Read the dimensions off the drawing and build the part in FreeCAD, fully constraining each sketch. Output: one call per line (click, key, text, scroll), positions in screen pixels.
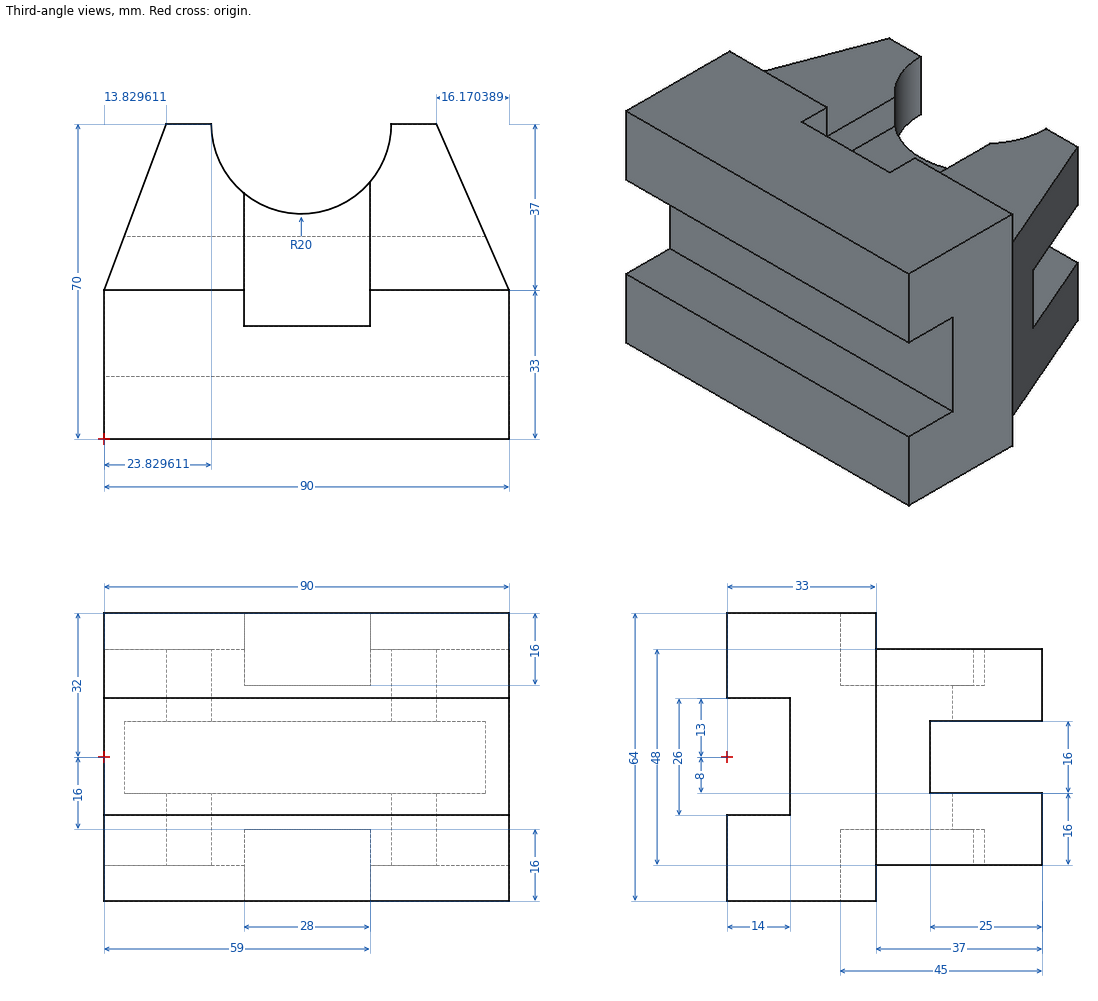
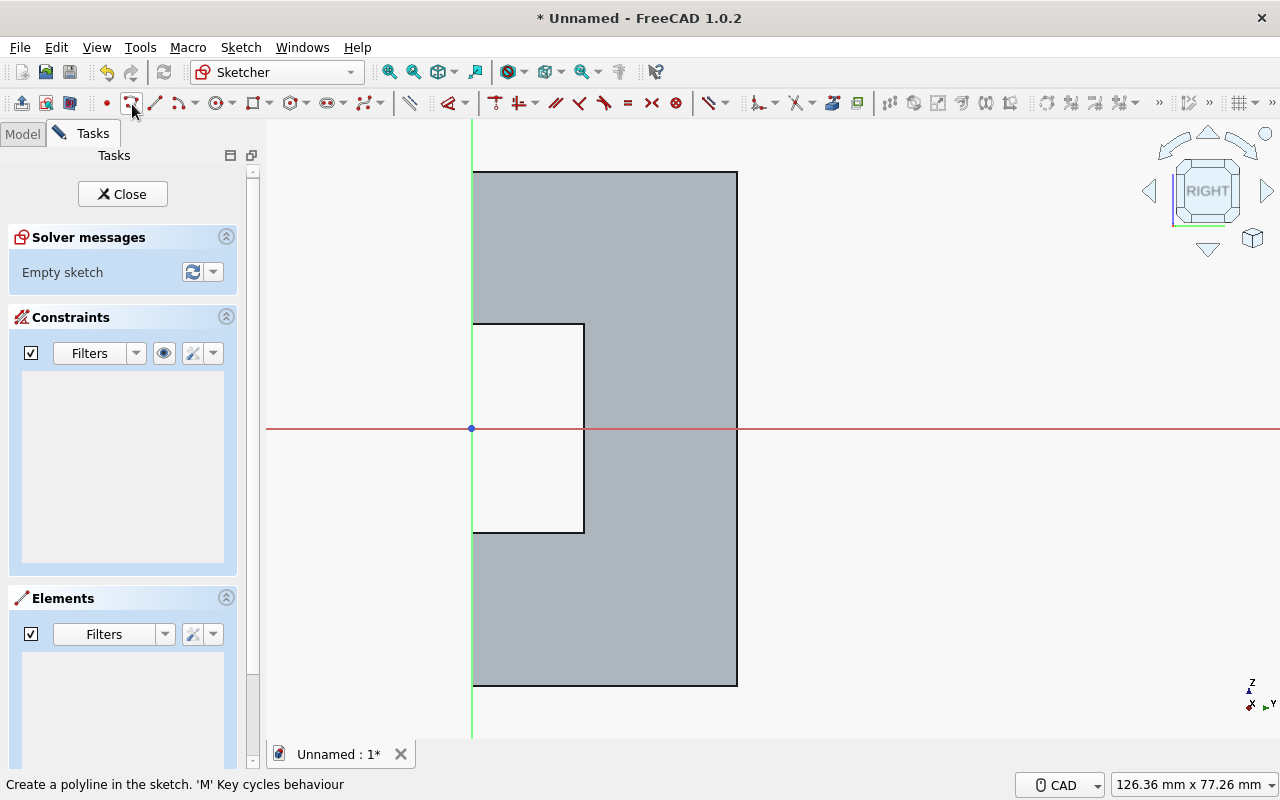
click(737, 236)
click(737, 621)
click(1034, 621)
click(1034, 493)
click(833, 493)
click(833, 365)
click(1034, 365)
click(1034, 236)
click(737, 237)
key(Escape)
key(Escape)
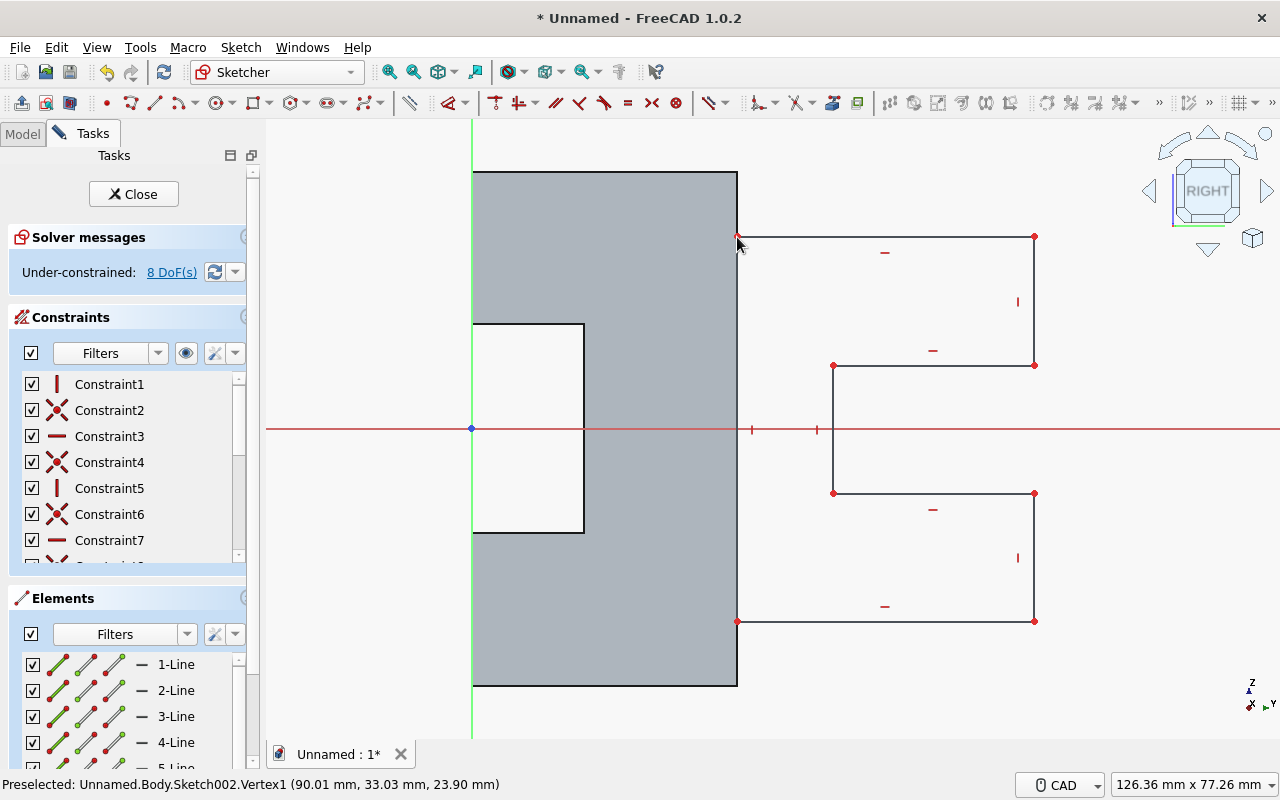
key(d)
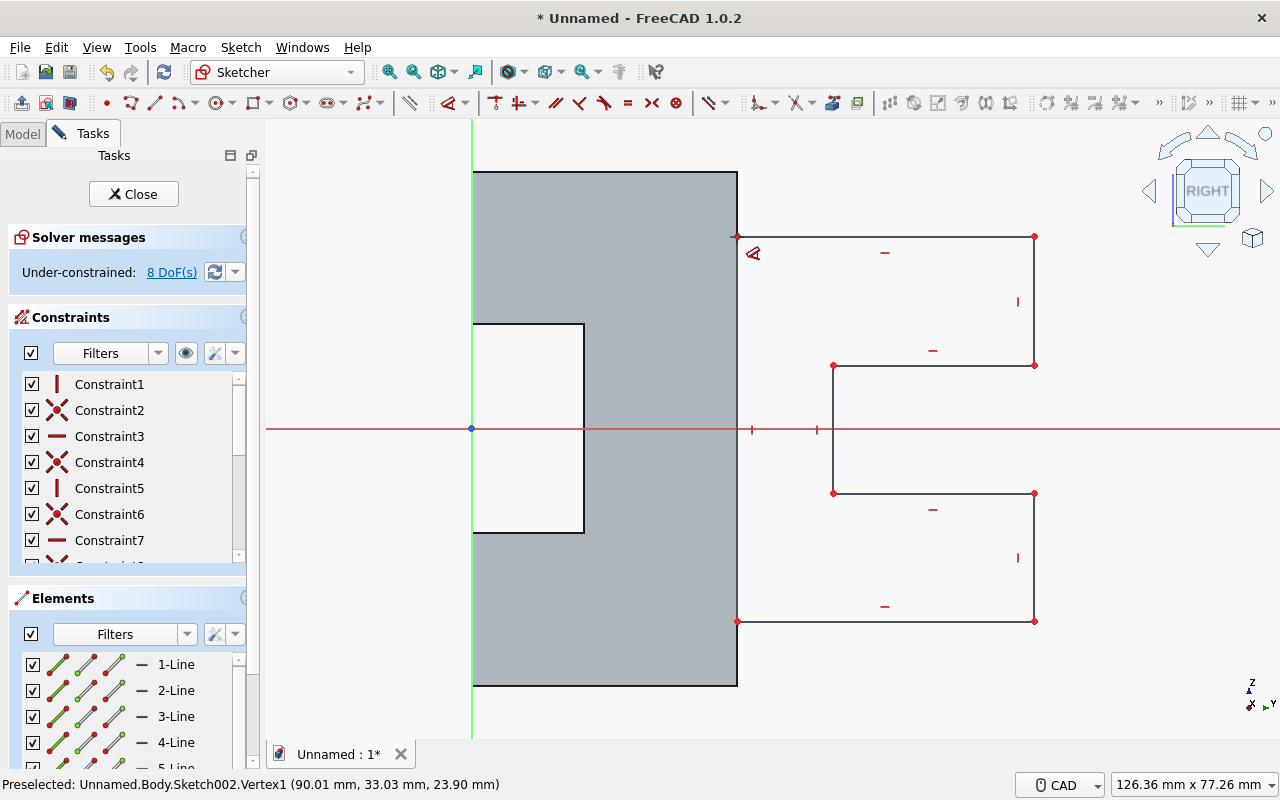
click(737, 353)
click(703, 341)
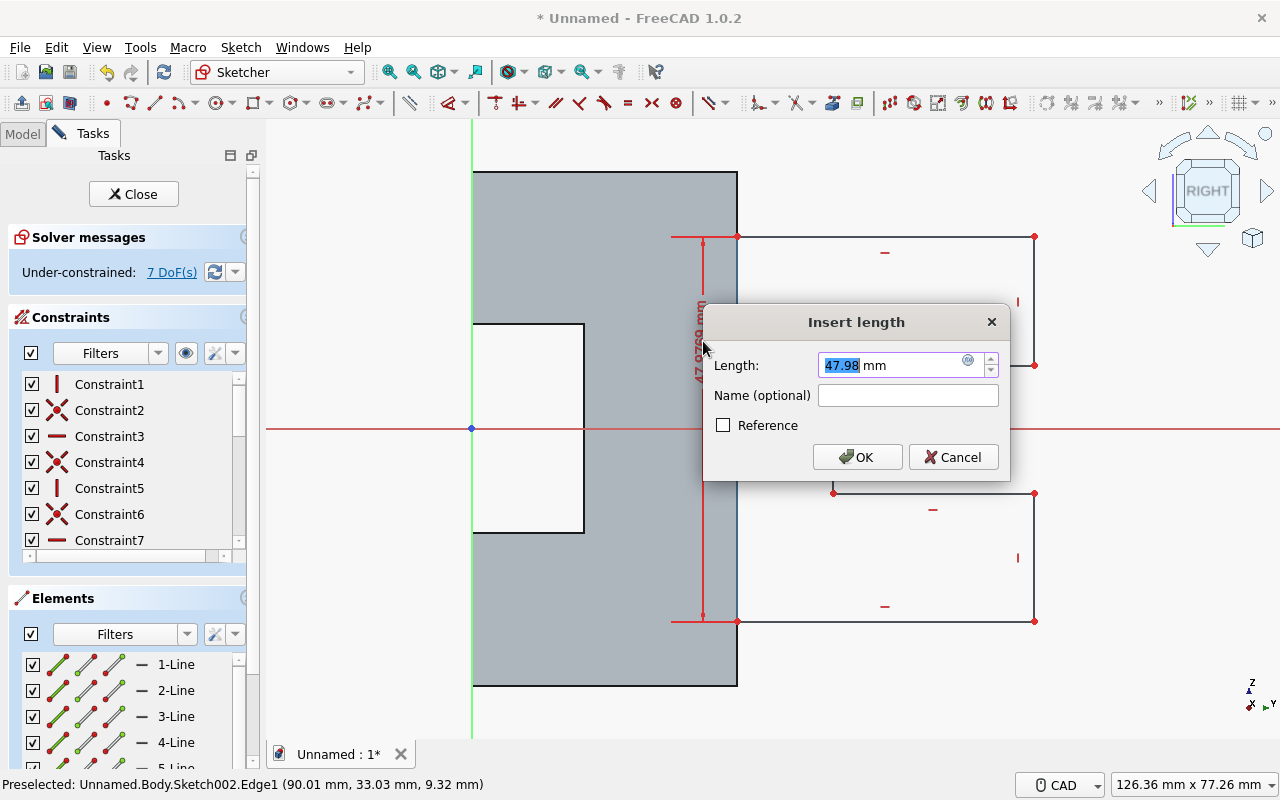
text(48)
key(Return)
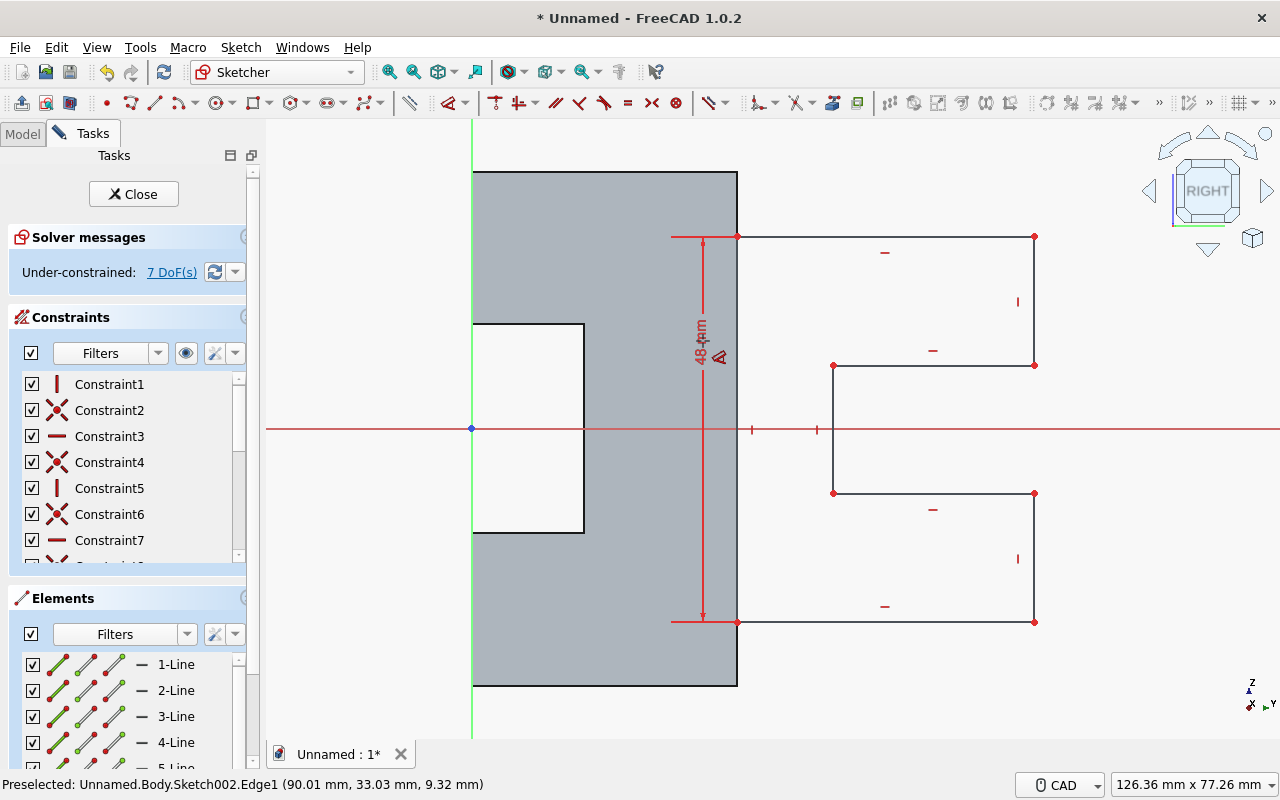
click(826, 622)
click(886, 656)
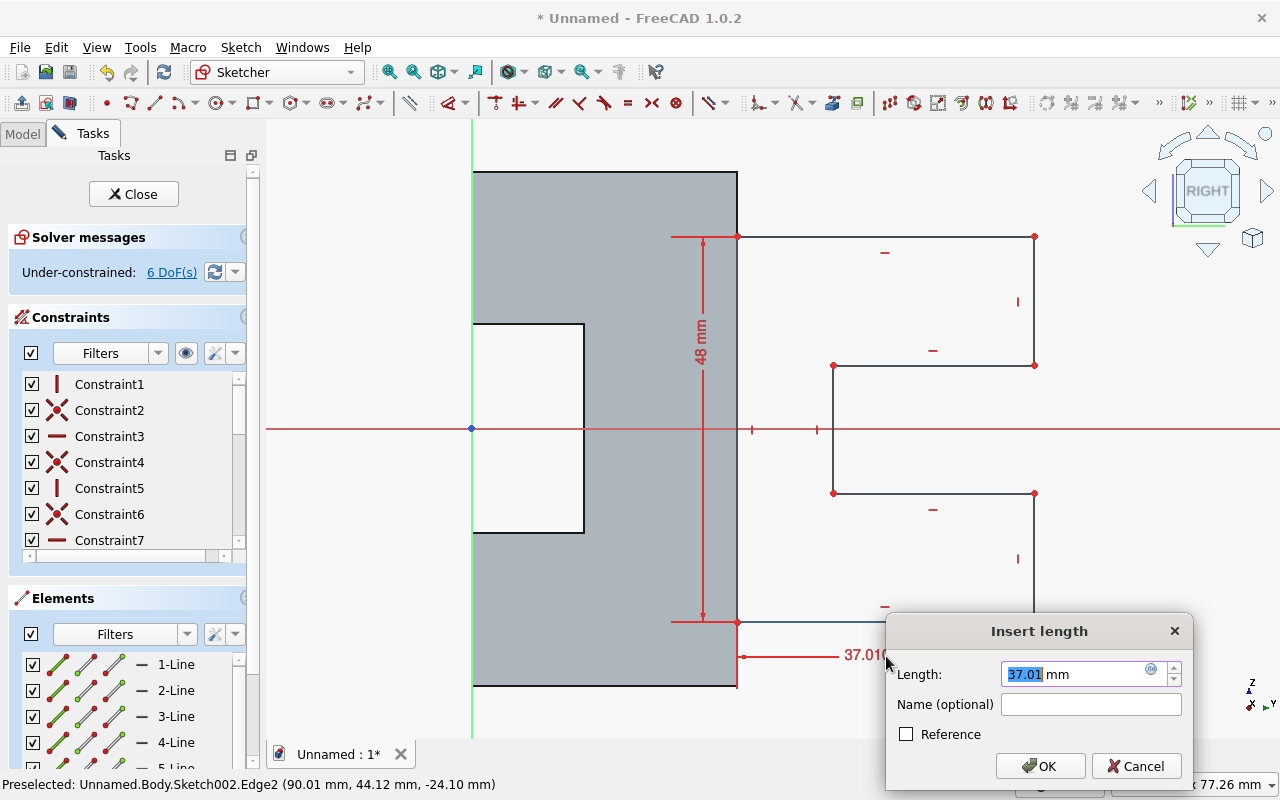
text(37)
key(Return)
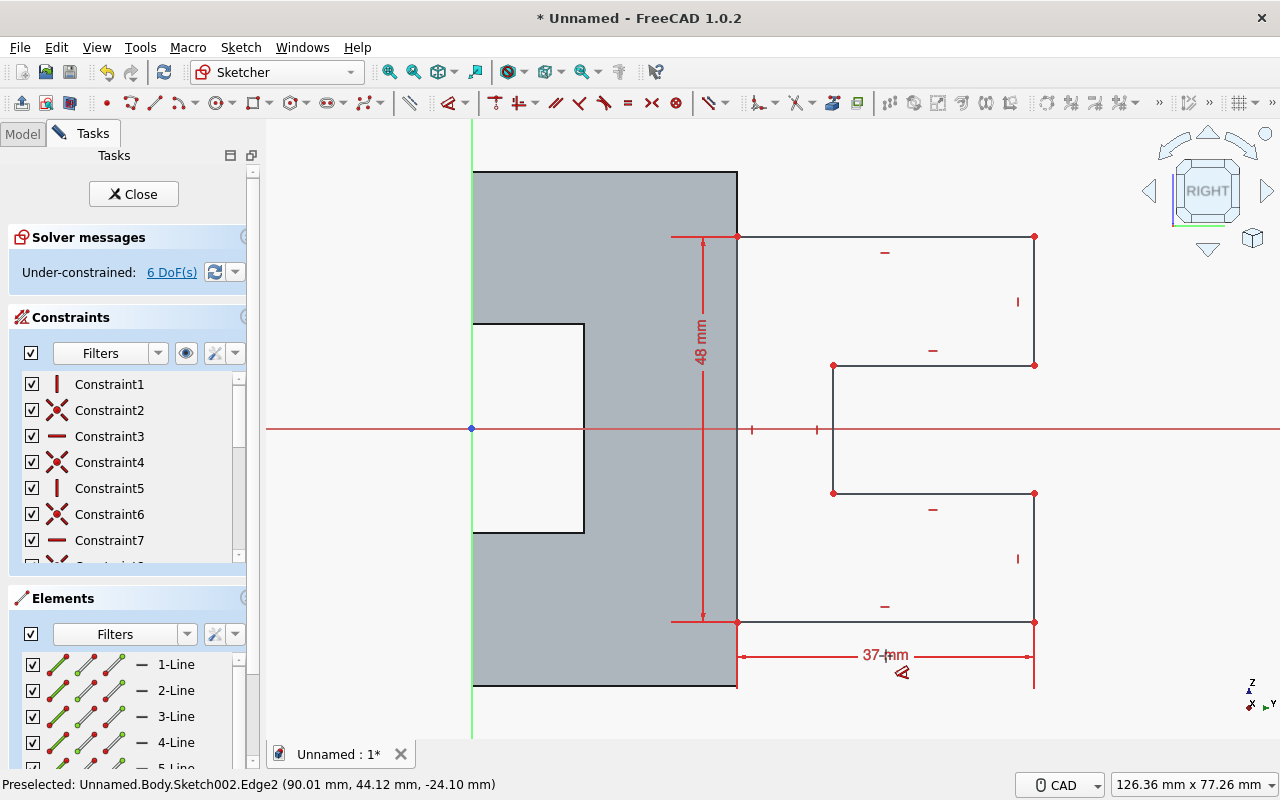
click(1034, 584)
click(1068, 558)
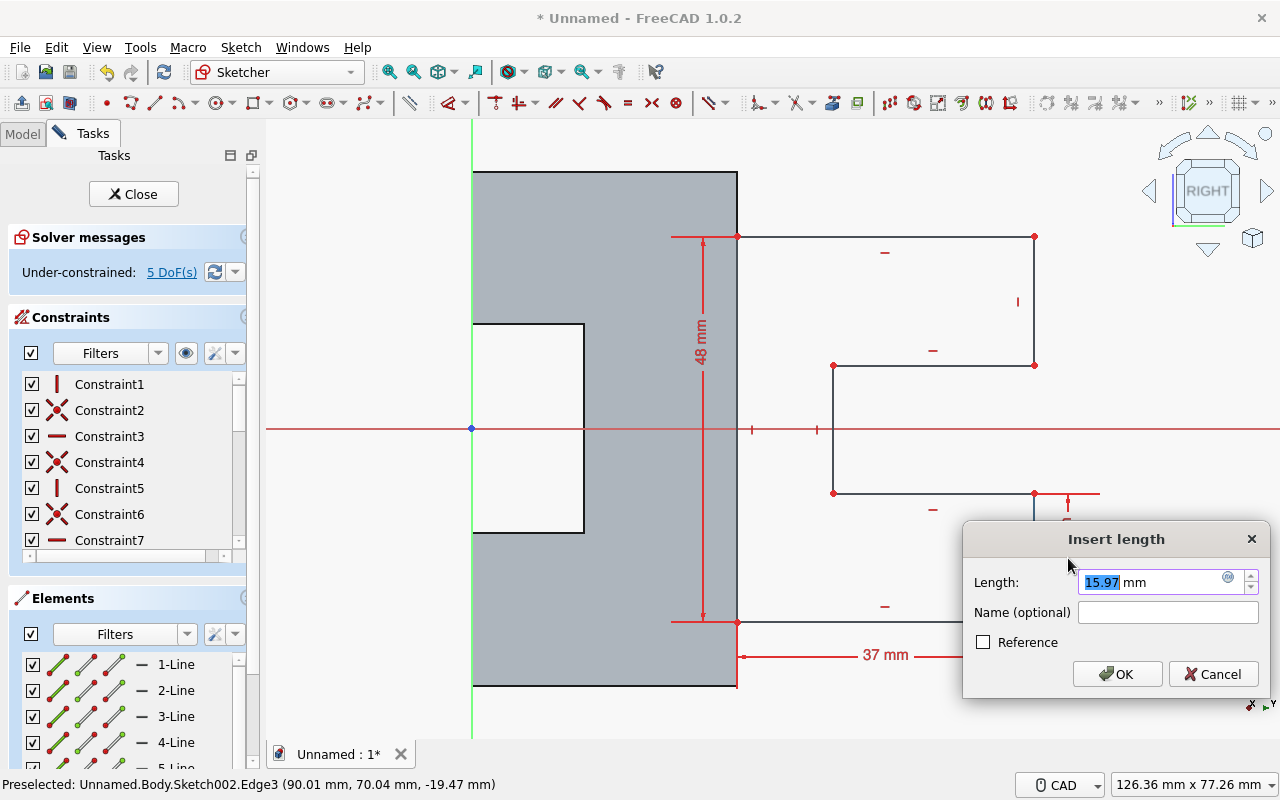
text(16)
key(Return)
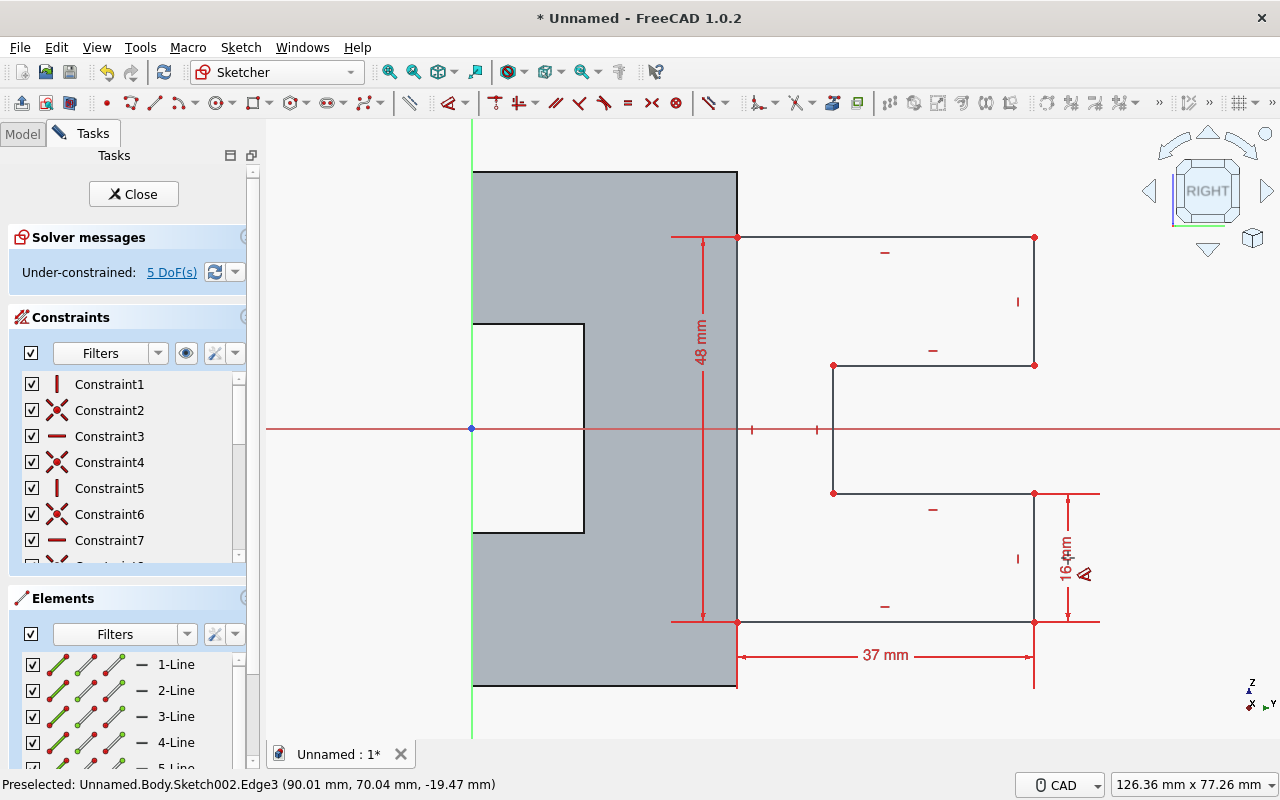
click(974, 494)
click(934, 528)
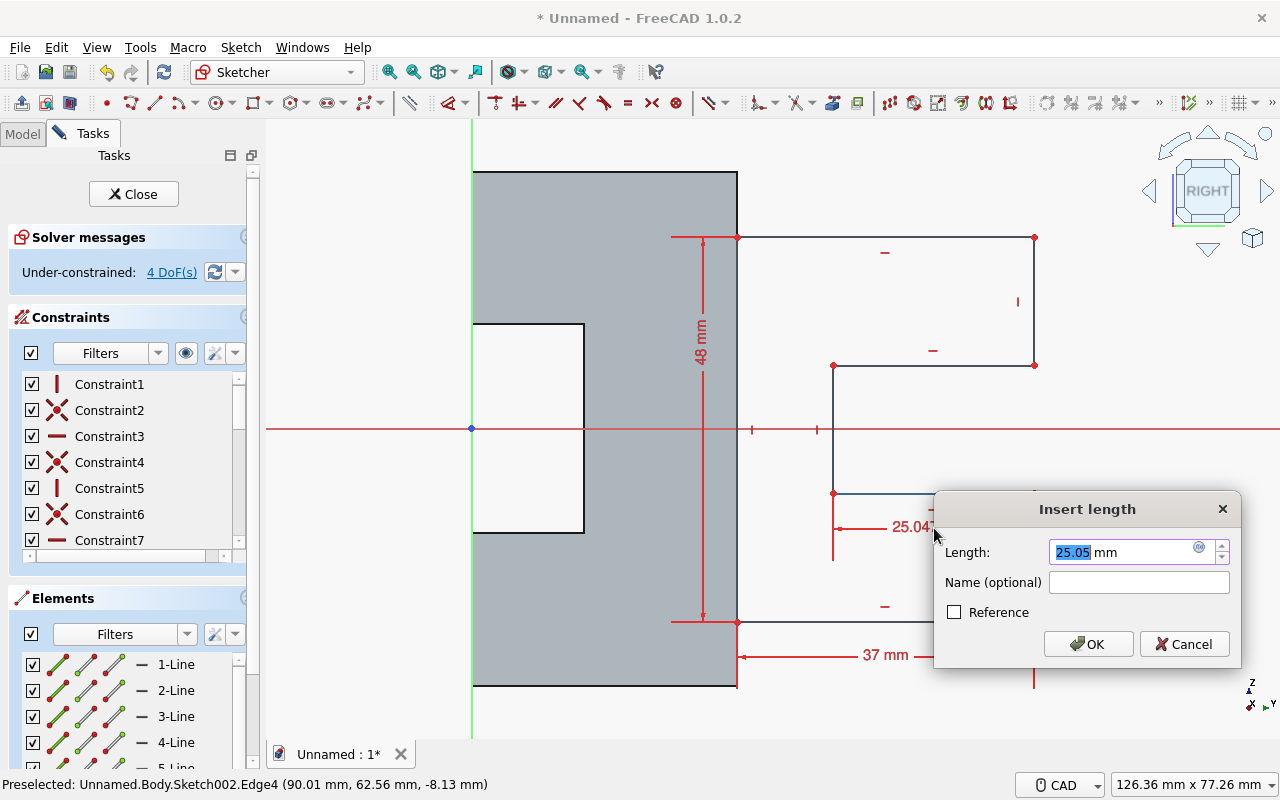
text(25)
key(Return)